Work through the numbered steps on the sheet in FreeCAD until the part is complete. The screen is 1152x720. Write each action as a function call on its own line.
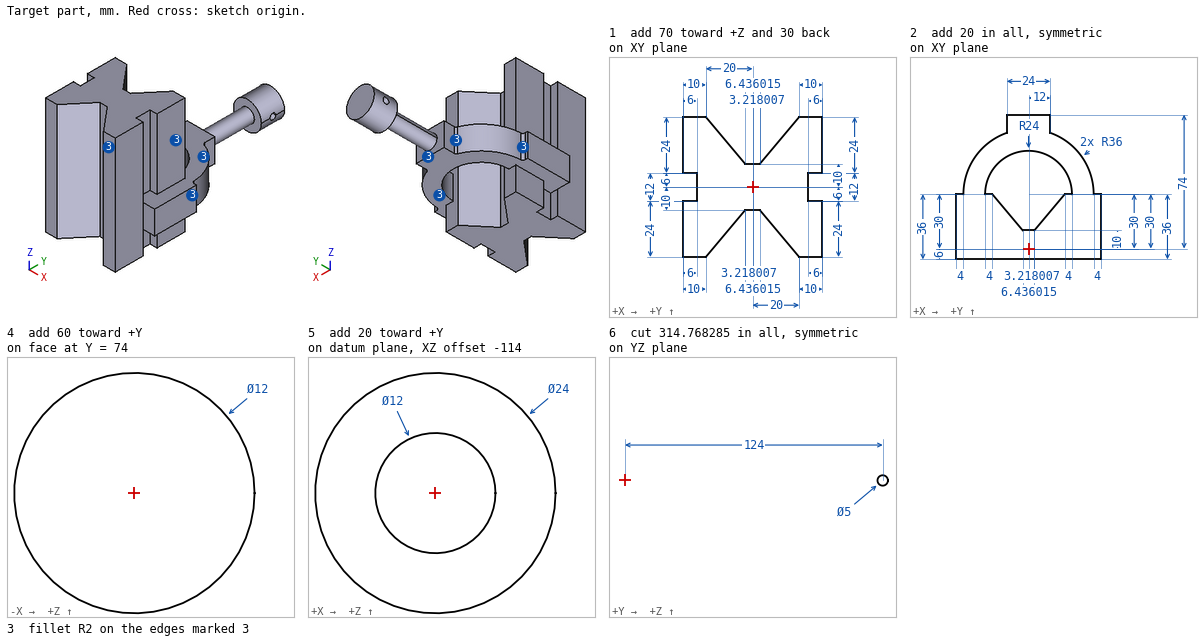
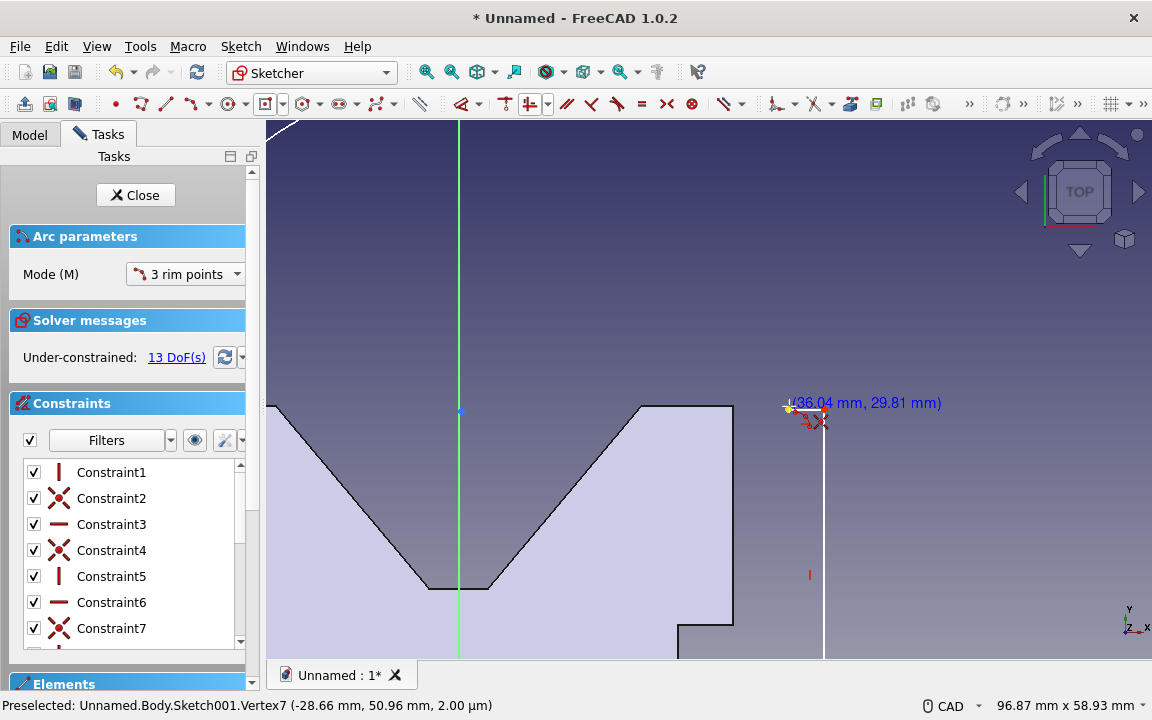
click(789, 410)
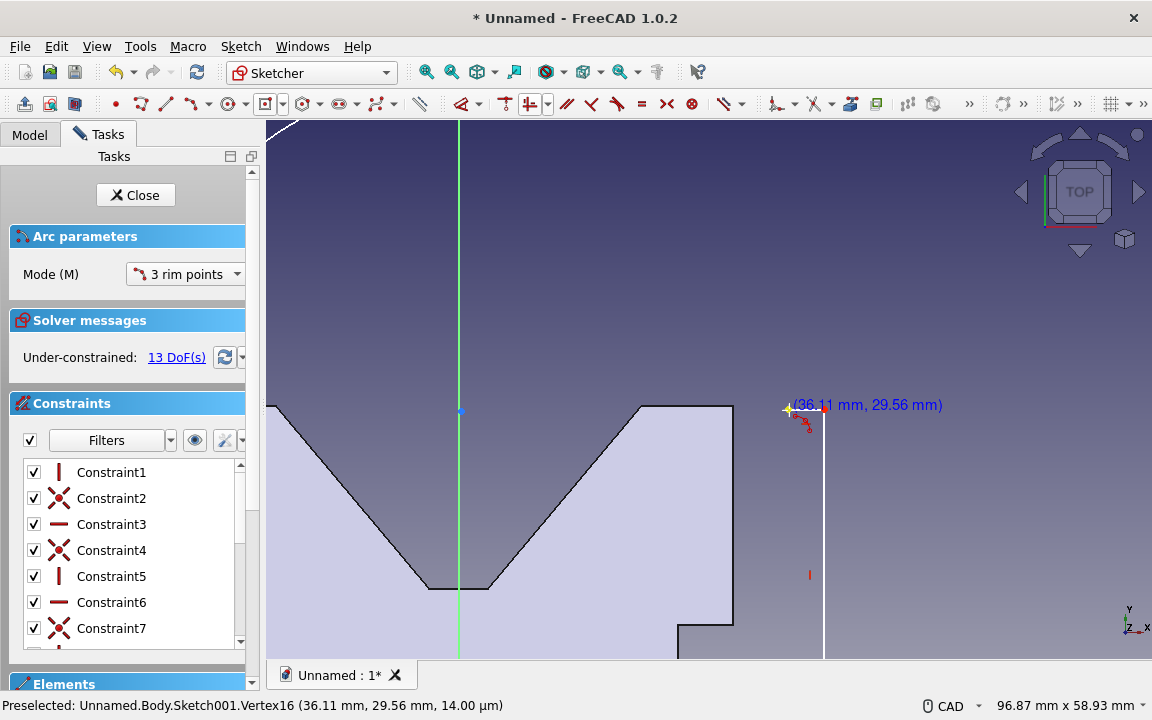
scroll(789, 406, down, 4)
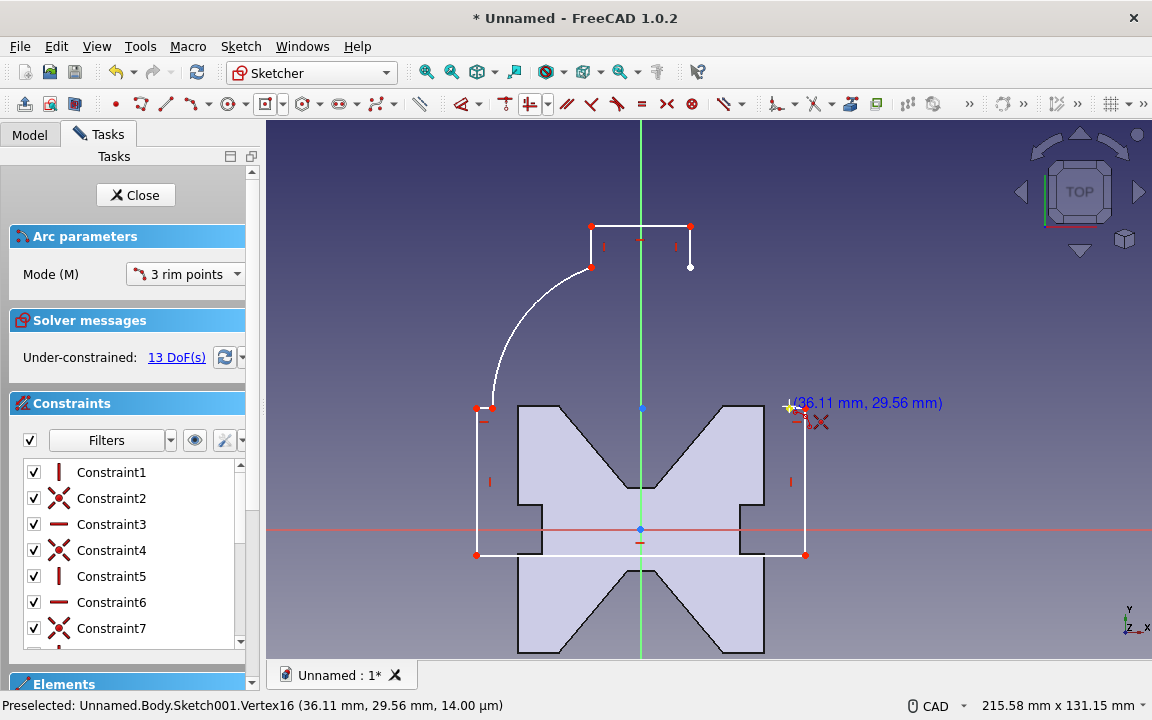
click(690, 268)
click(762, 321)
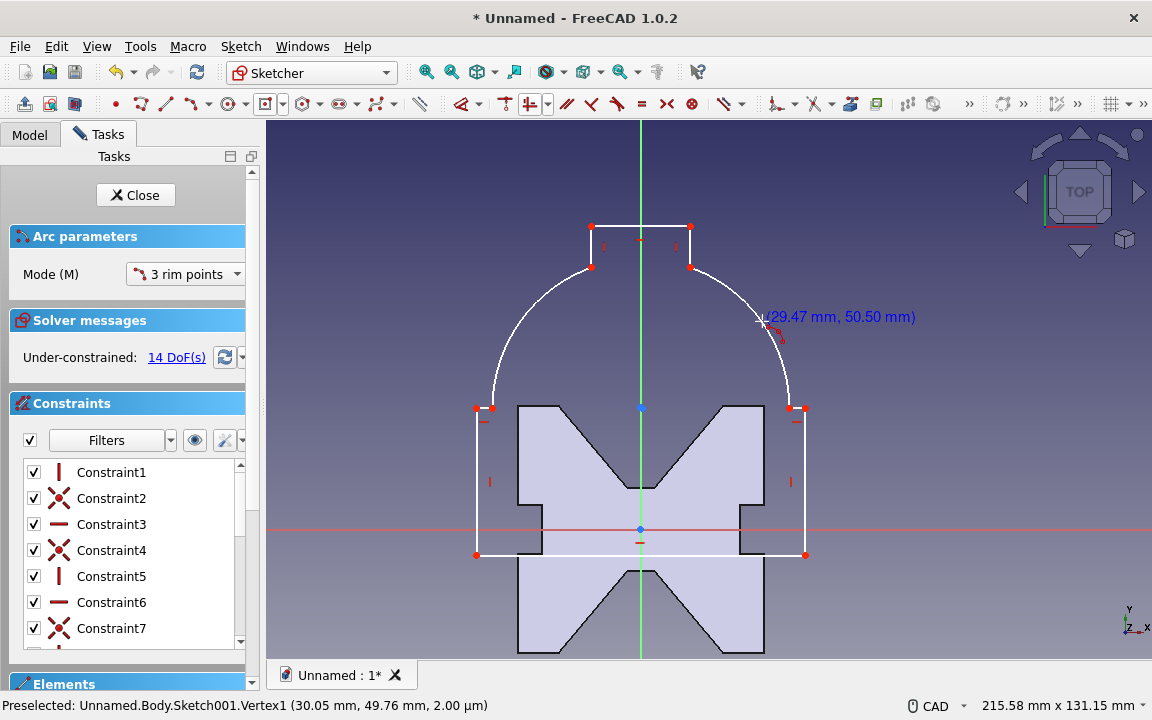
click(141, 104)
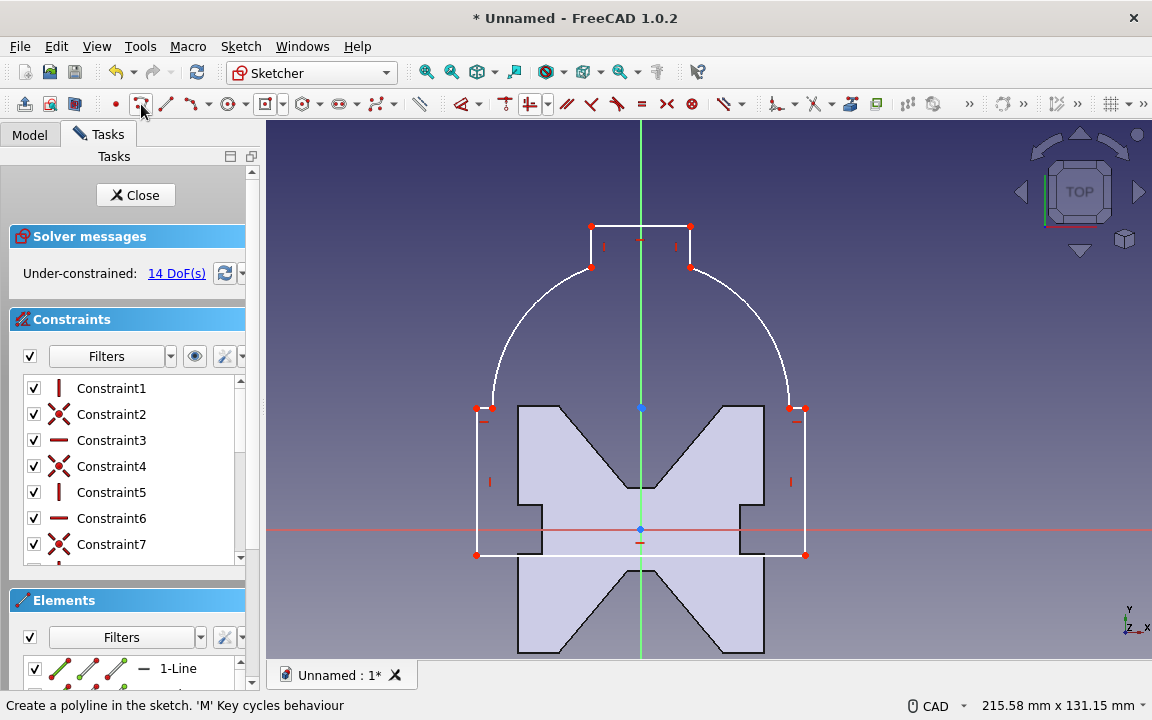
click(740, 406)
click(723, 406)
click(654, 488)
click(628, 488)
click(559, 406)
click(542, 406)
right_click(542, 406)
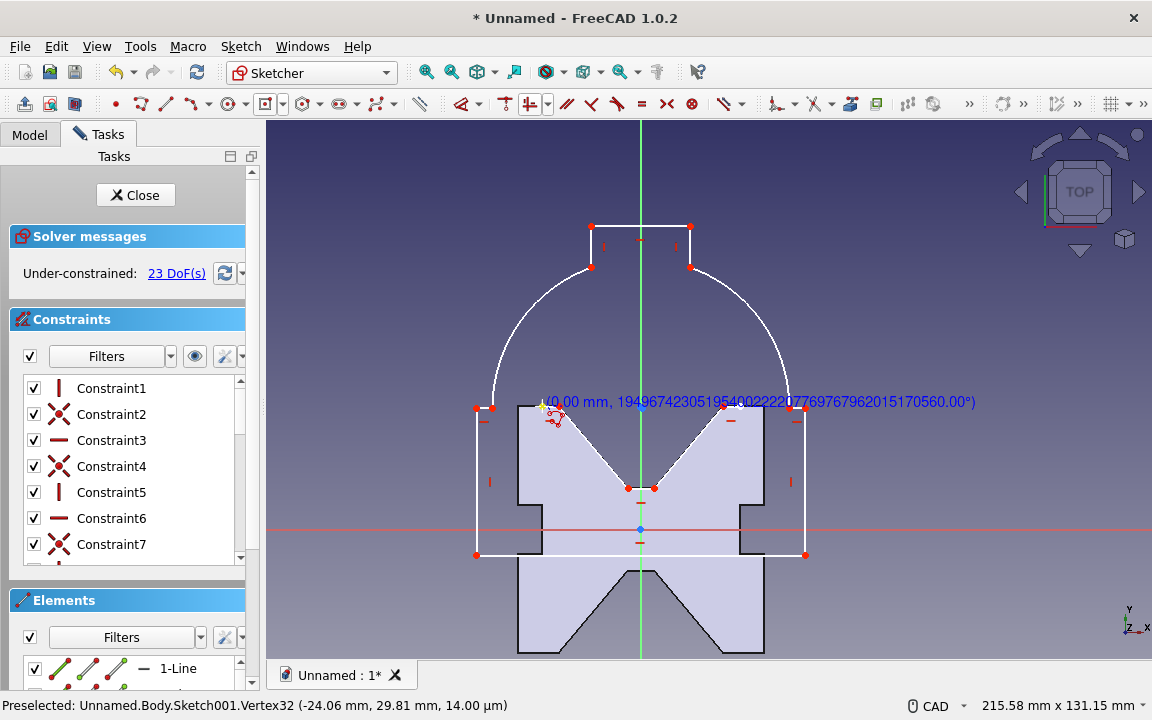
click(190, 104)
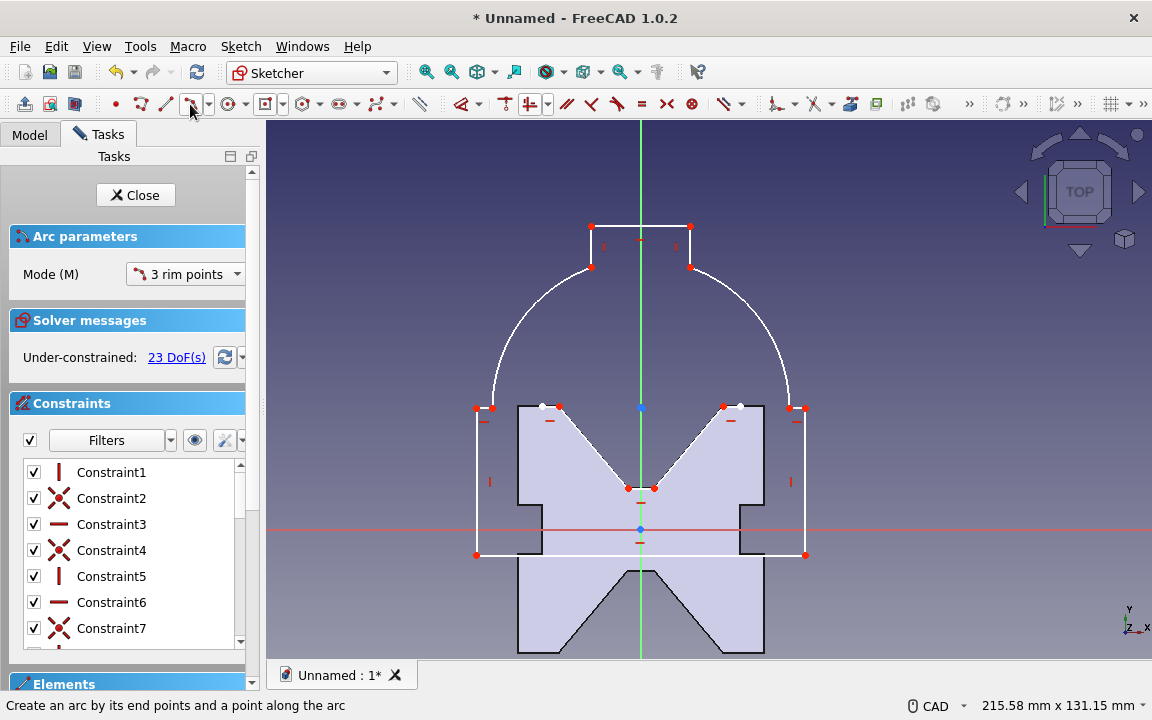
scroll(542, 406, up, 4)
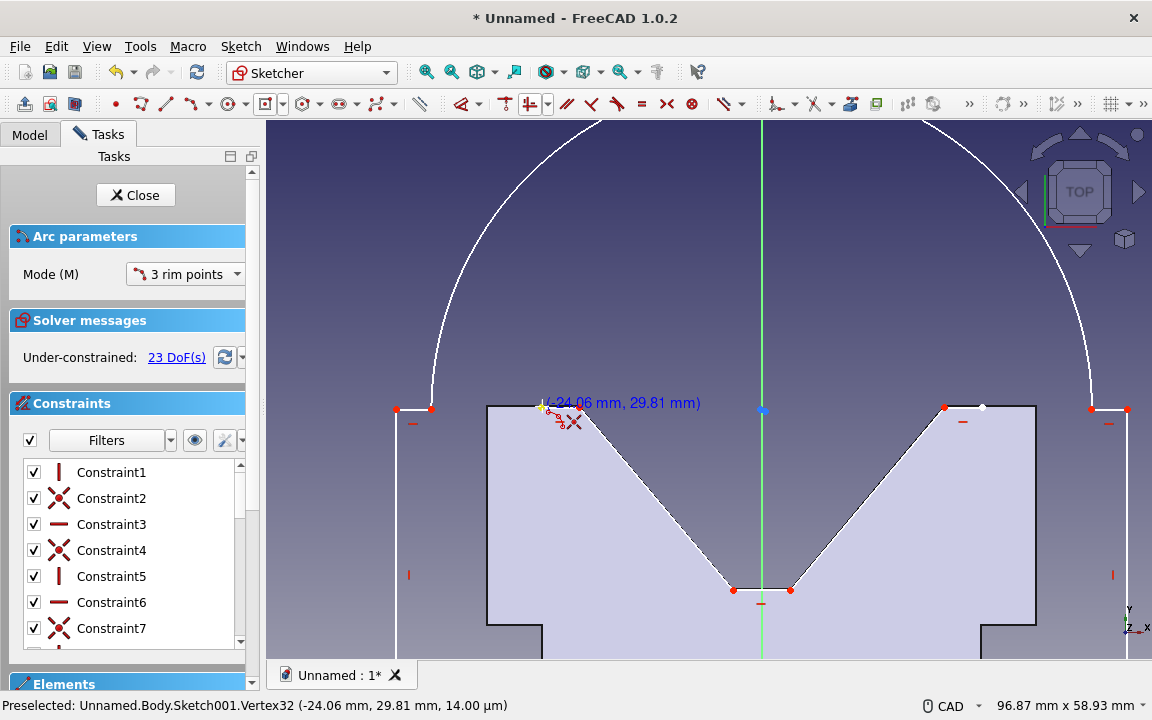
click(542, 408)
click(982, 408)
click(829, 197)
key(Escape)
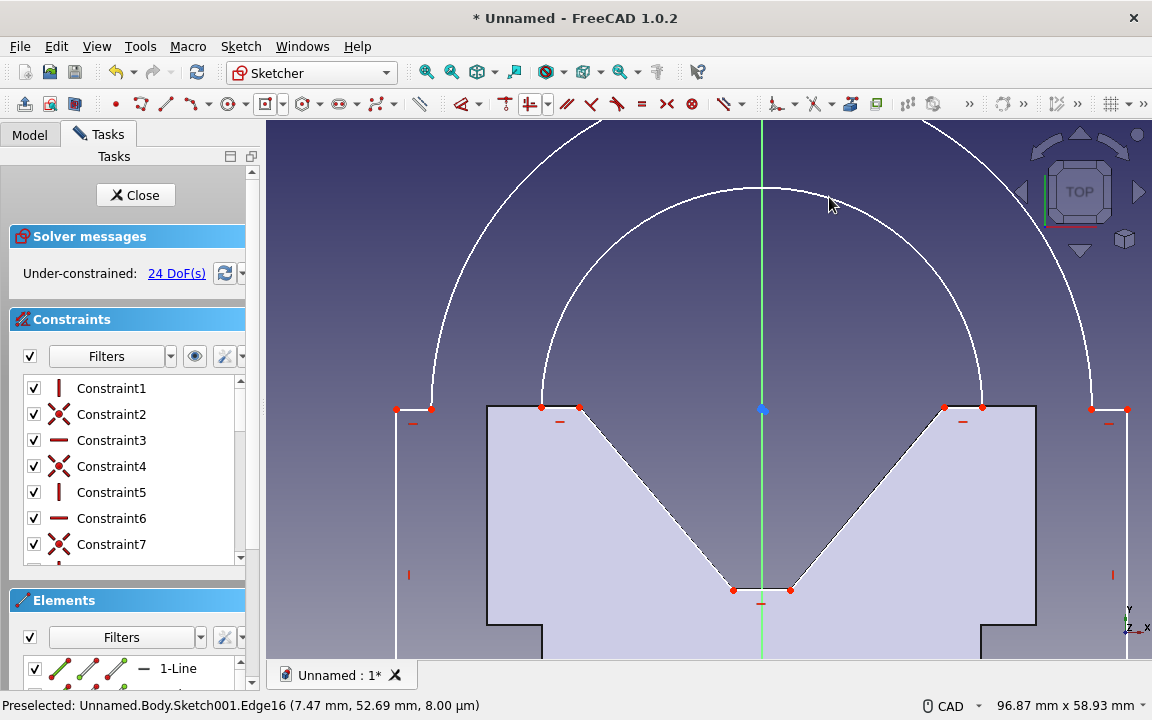
click(547, 159)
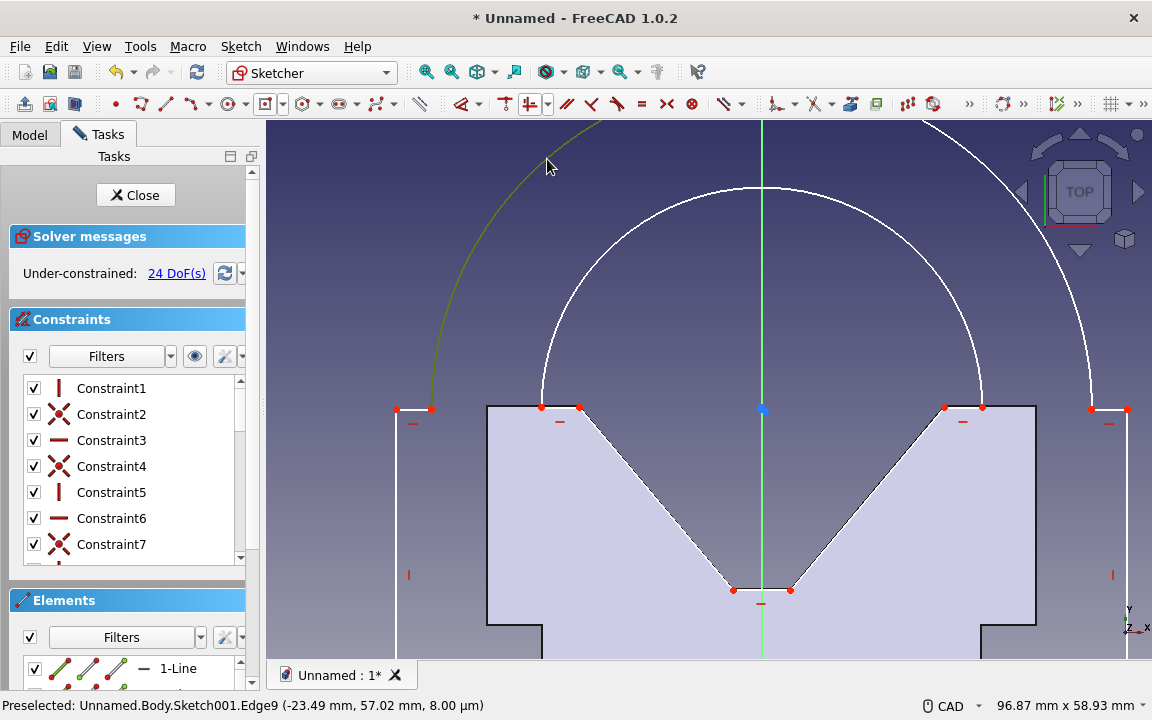
click(977, 158)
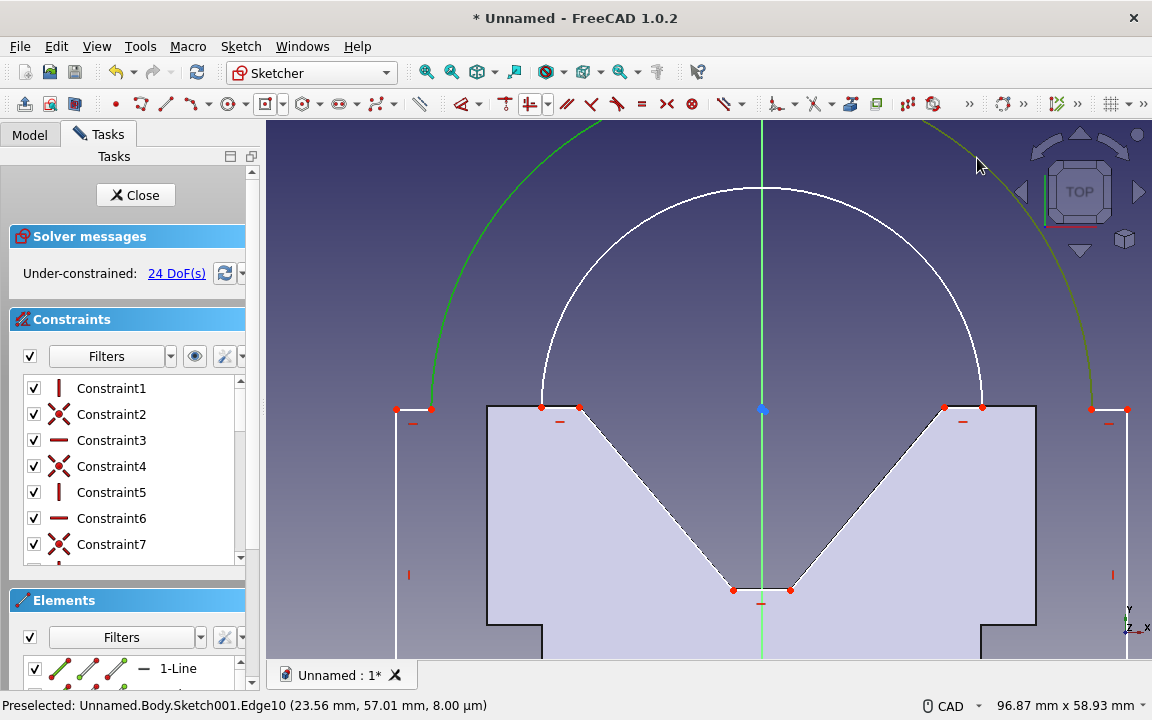
click(505, 104)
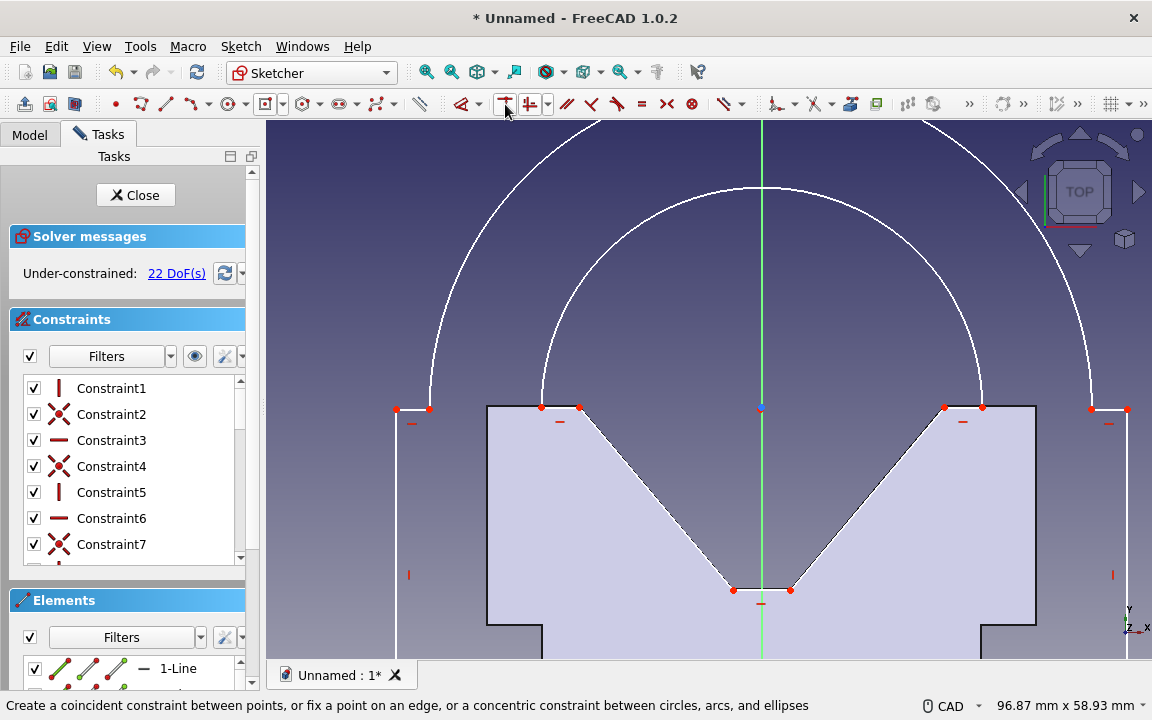
click(546, 158)